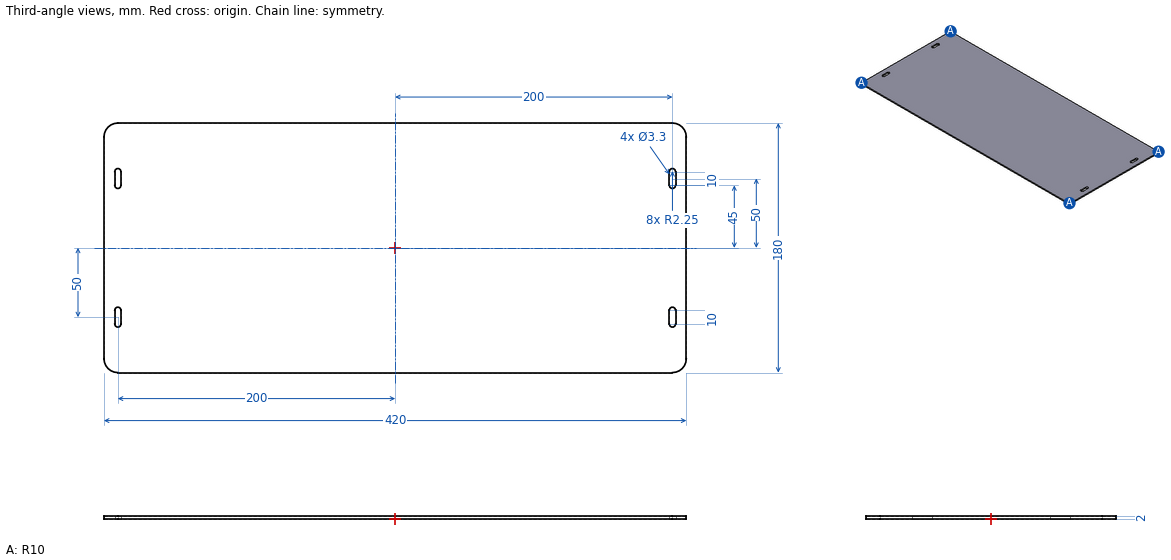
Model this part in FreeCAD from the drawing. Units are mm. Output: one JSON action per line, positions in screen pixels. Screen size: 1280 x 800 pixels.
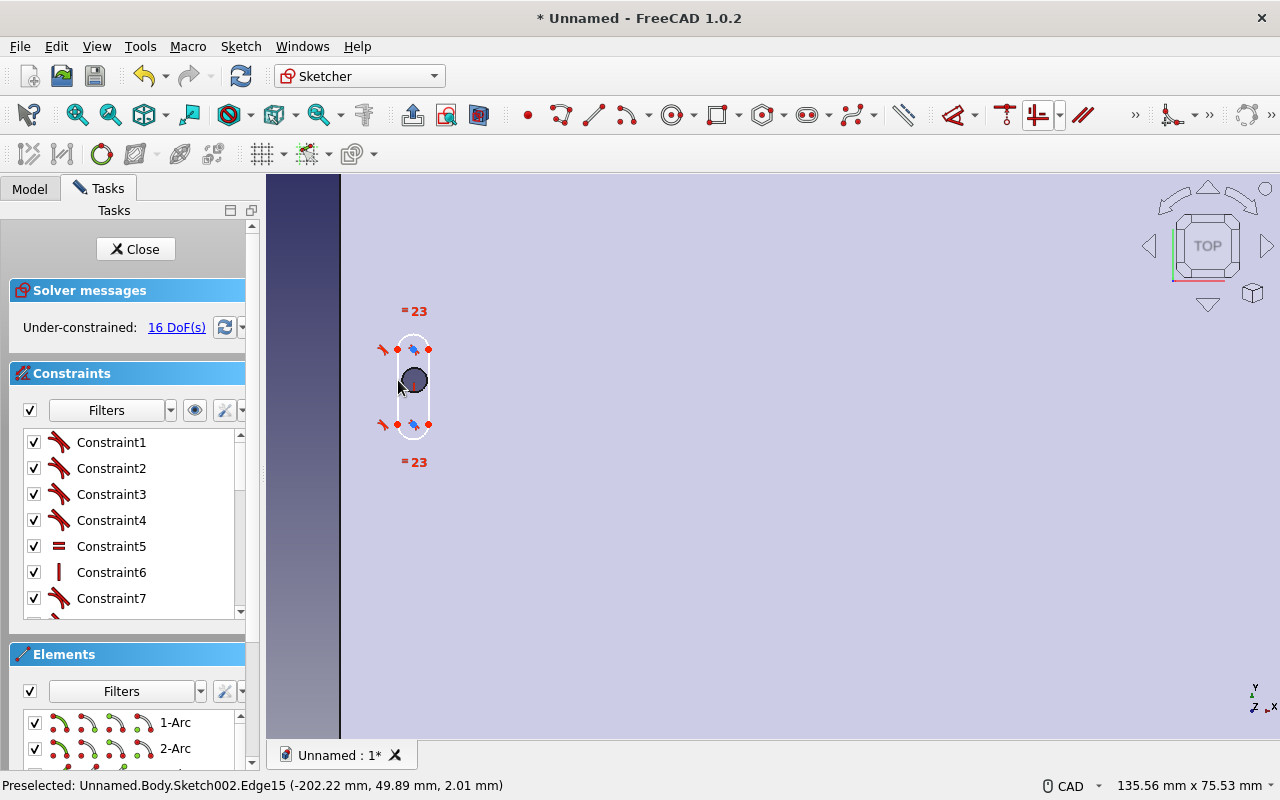
{"action": "scroll", "coordinate": [399, 381], "scroll_direction": "down", "scroll_amount": 8}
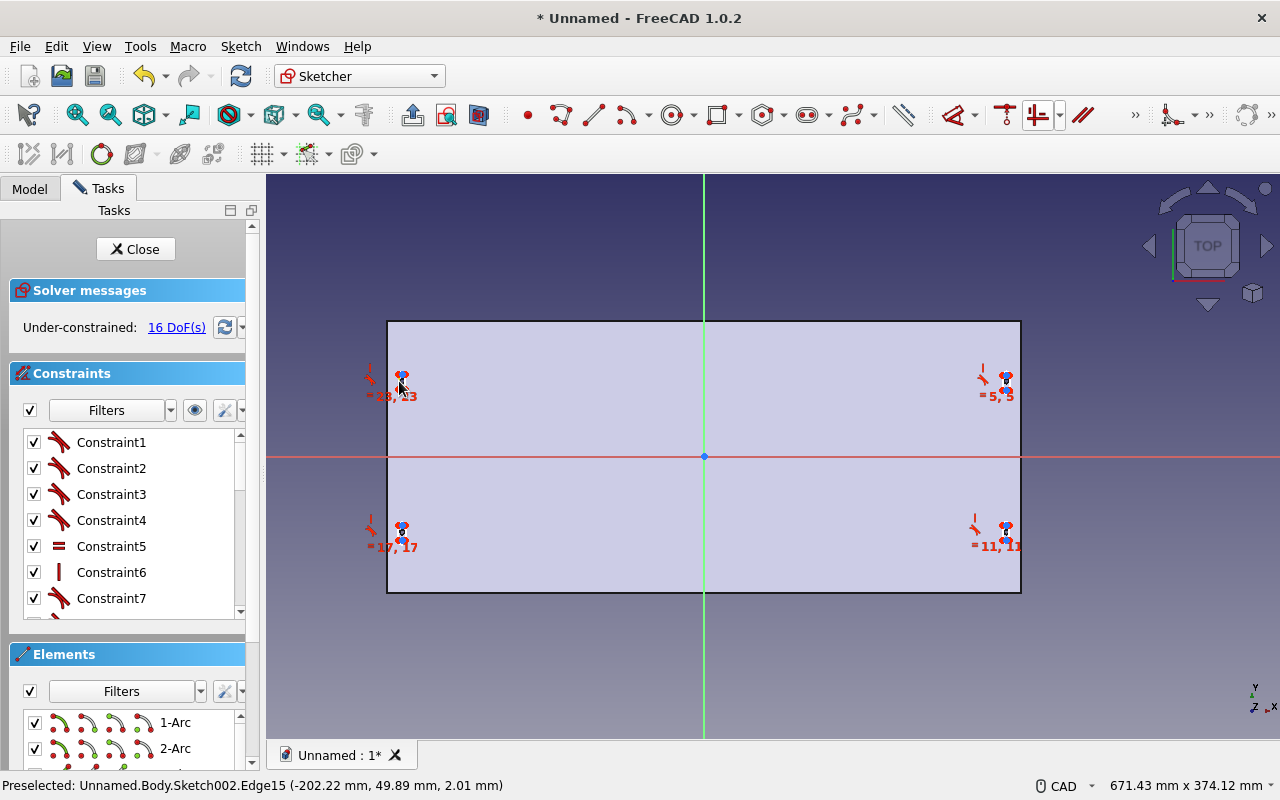
{"action": "scroll", "coordinate": [1004, 393], "scroll_direction": "up", "scroll_amount": 8}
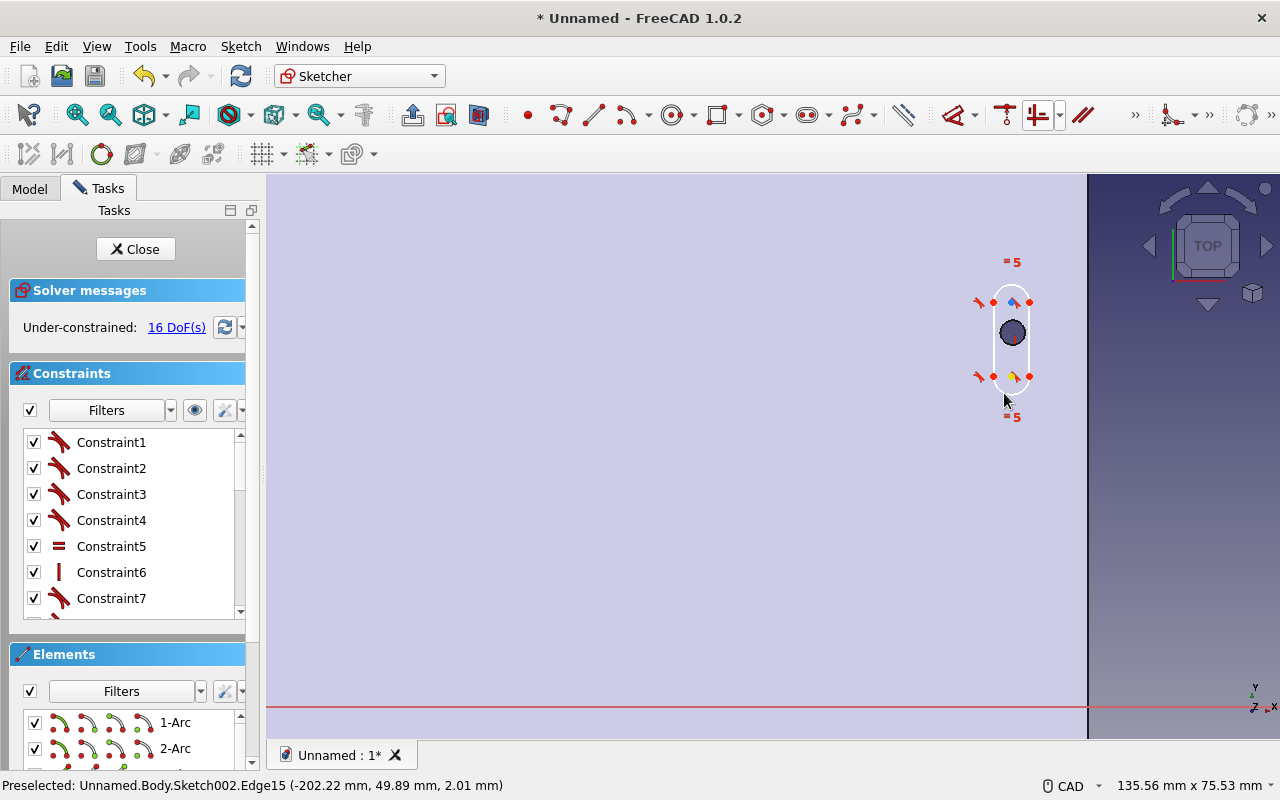
{"action": "left_click", "coordinate": [1001, 391]}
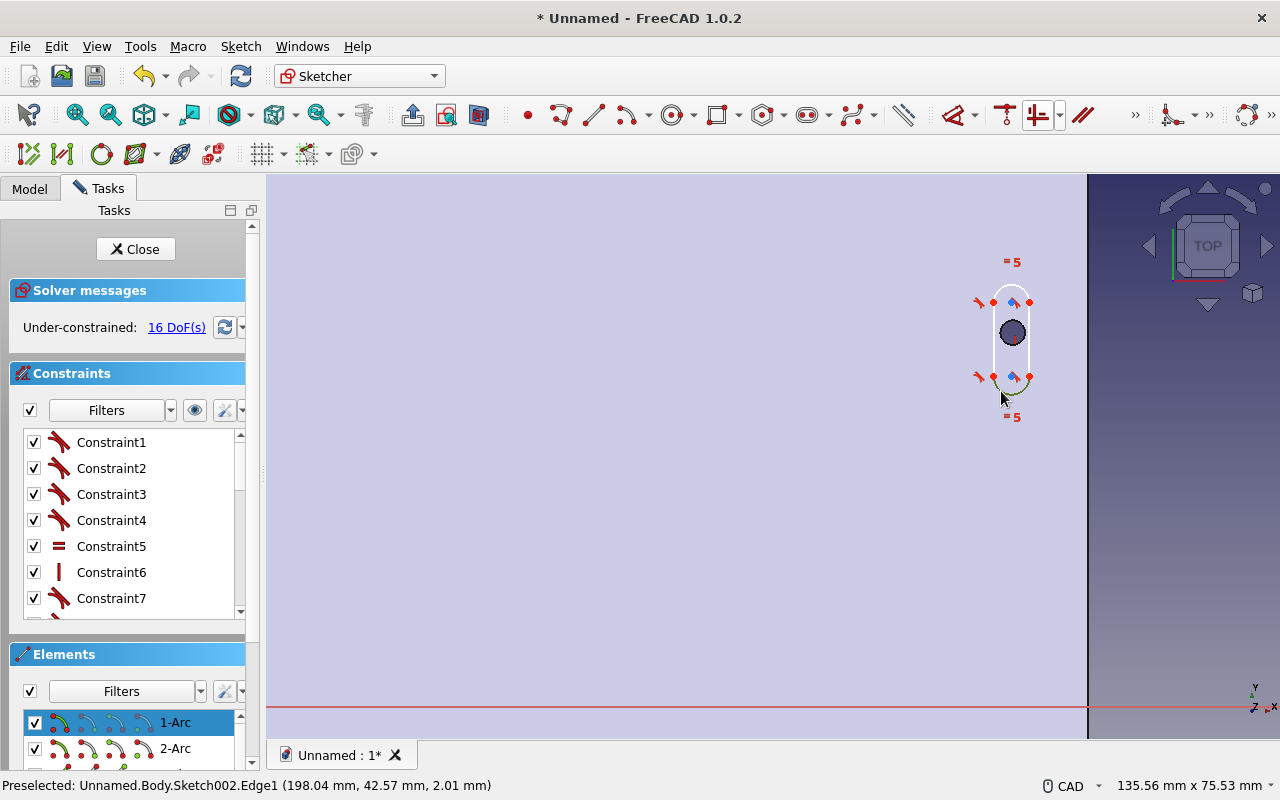
{"action": "scroll", "coordinate": [1005, 393], "scroll_direction": "down", "scroll_amount": 8}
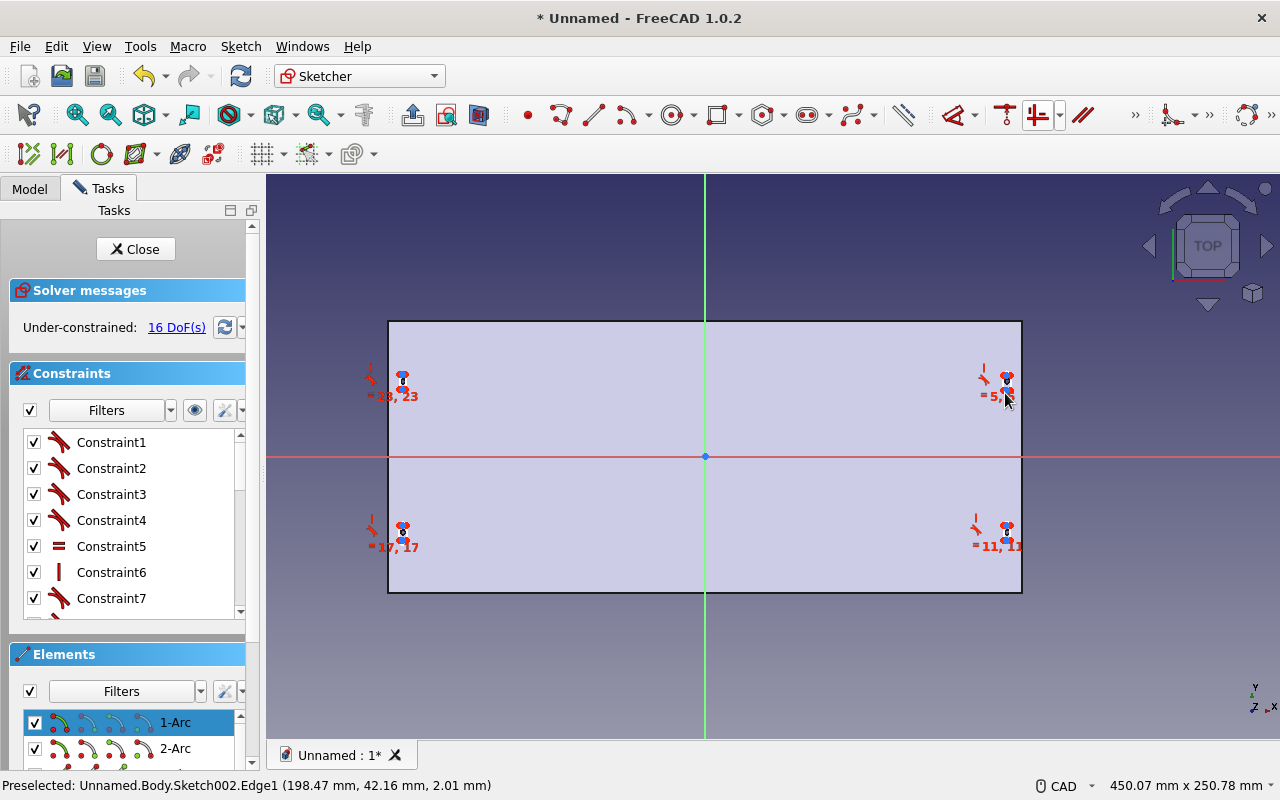
{"action": "scroll", "coordinate": [1005, 543], "scroll_direction": "up", "scroll_amount": 8}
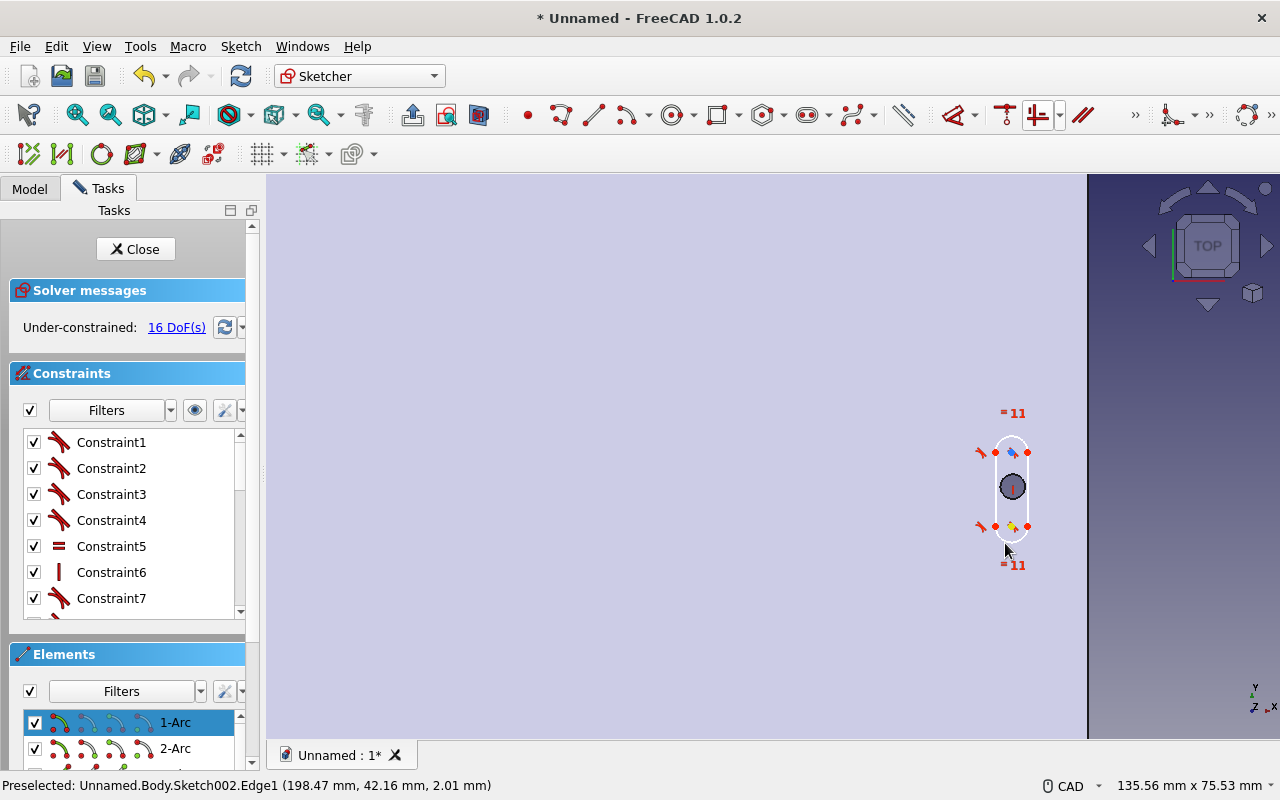
{"action": "left_click", "coordinate": [1002, 539]}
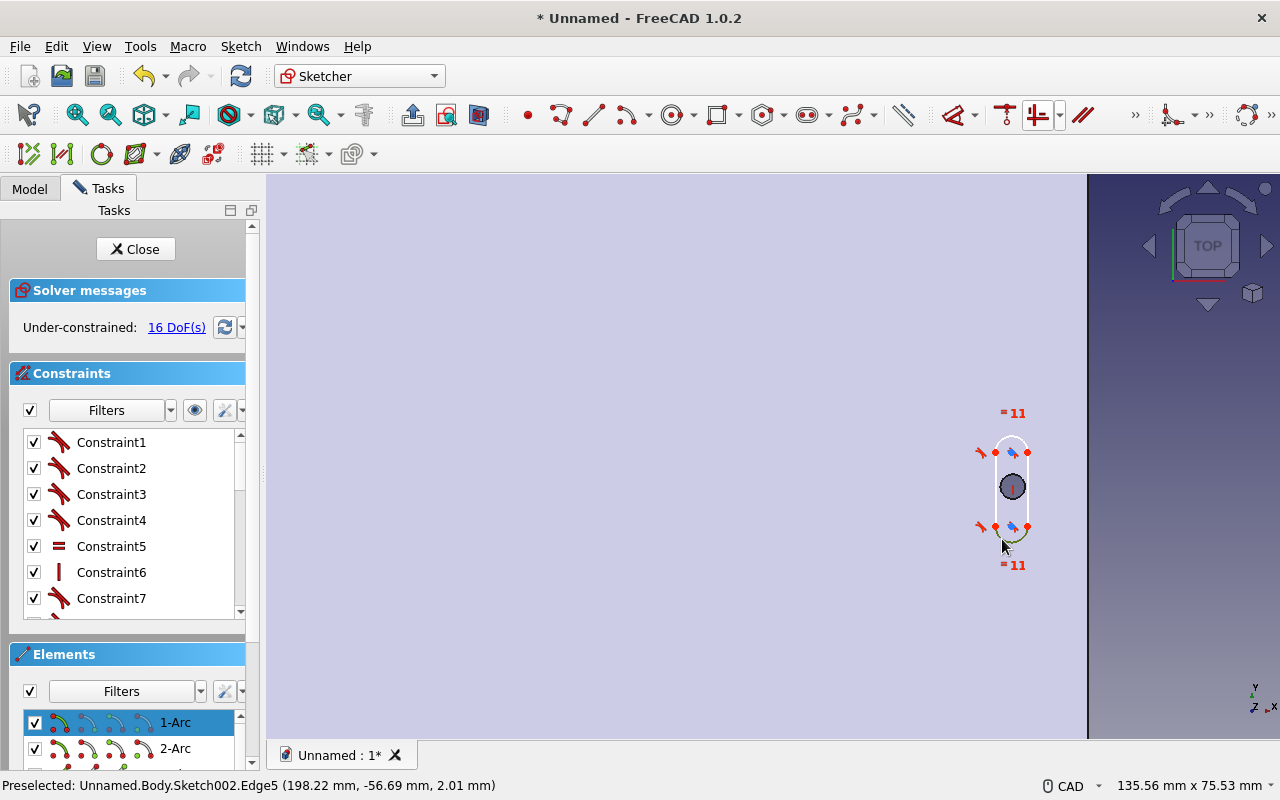
{"action": "scroll", "coordinate": [1005, 543], "scroll_direction": "down", "scroll_amount": 8}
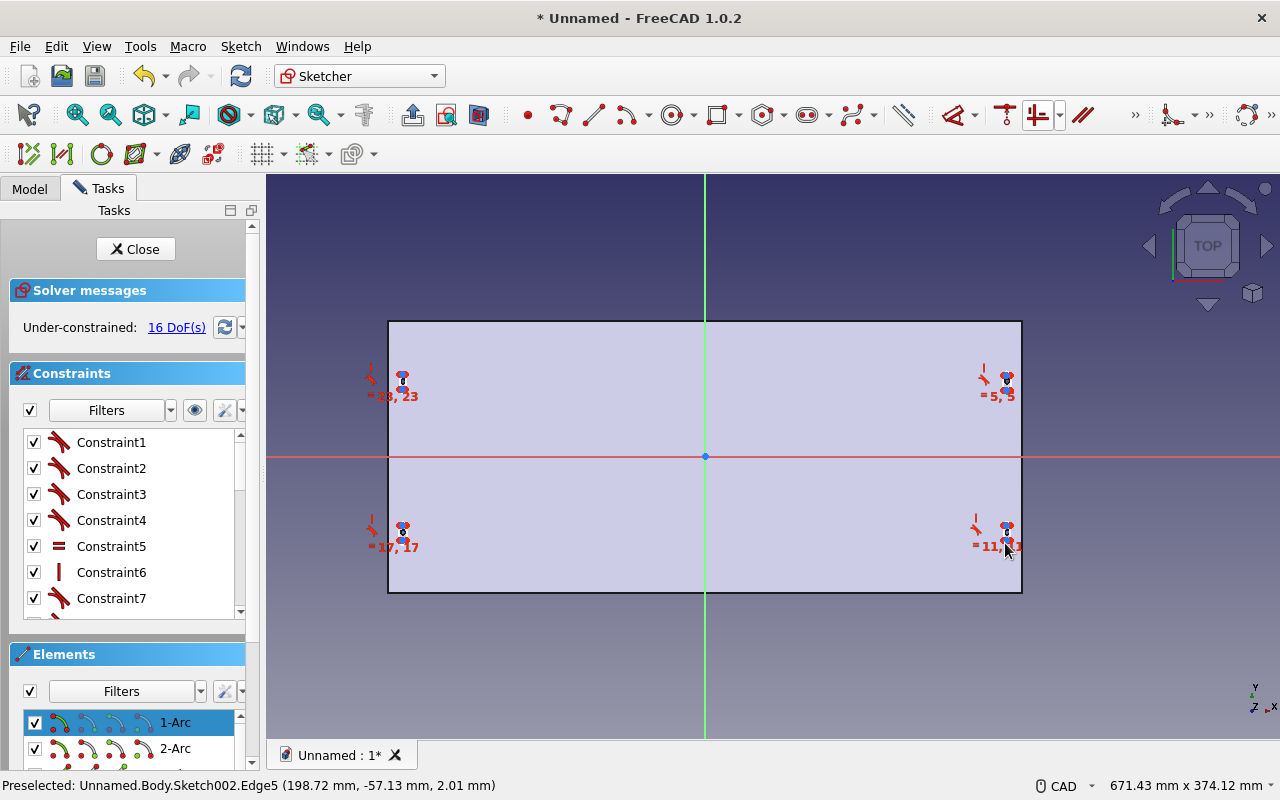
{"action": "scroll", "coordinate": [401, 544], "scroll_direction": "up", "scroll_amount": 8}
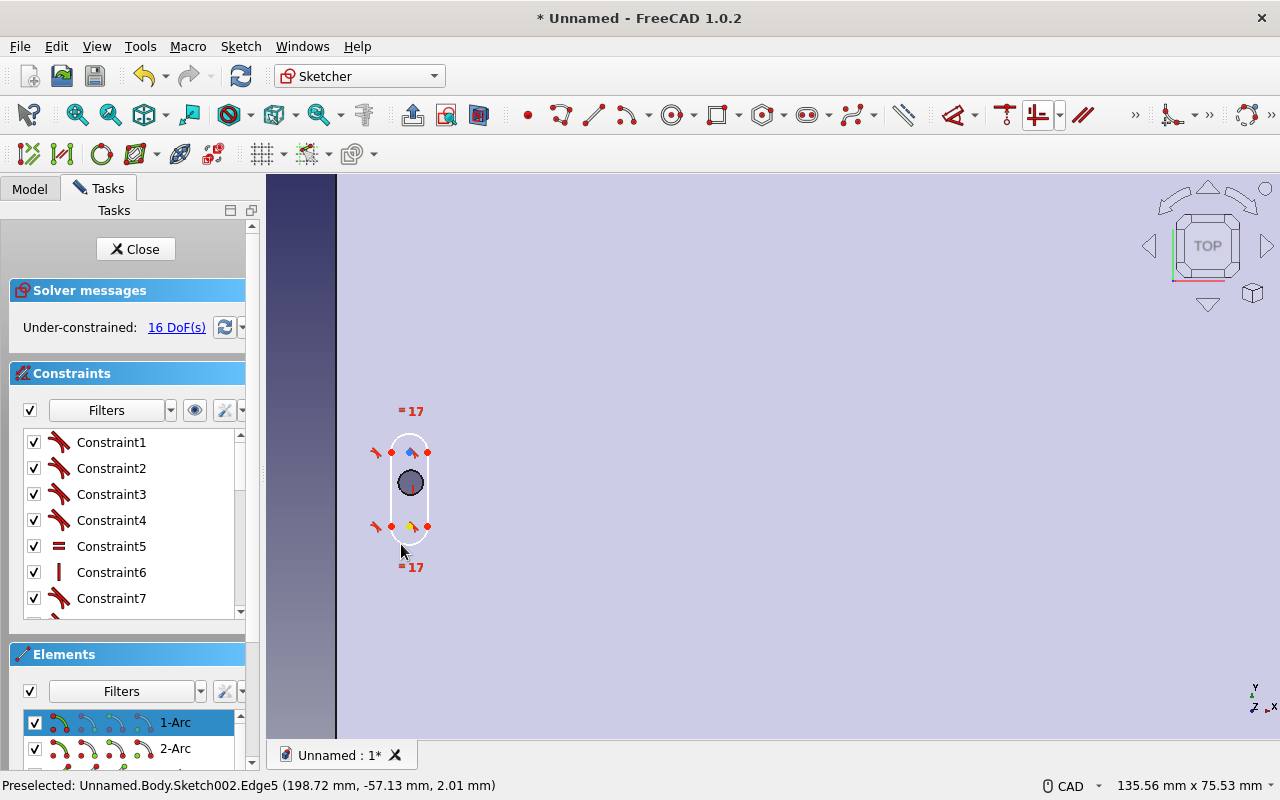
{"action": "left_click", "coordinate": [399, 541]}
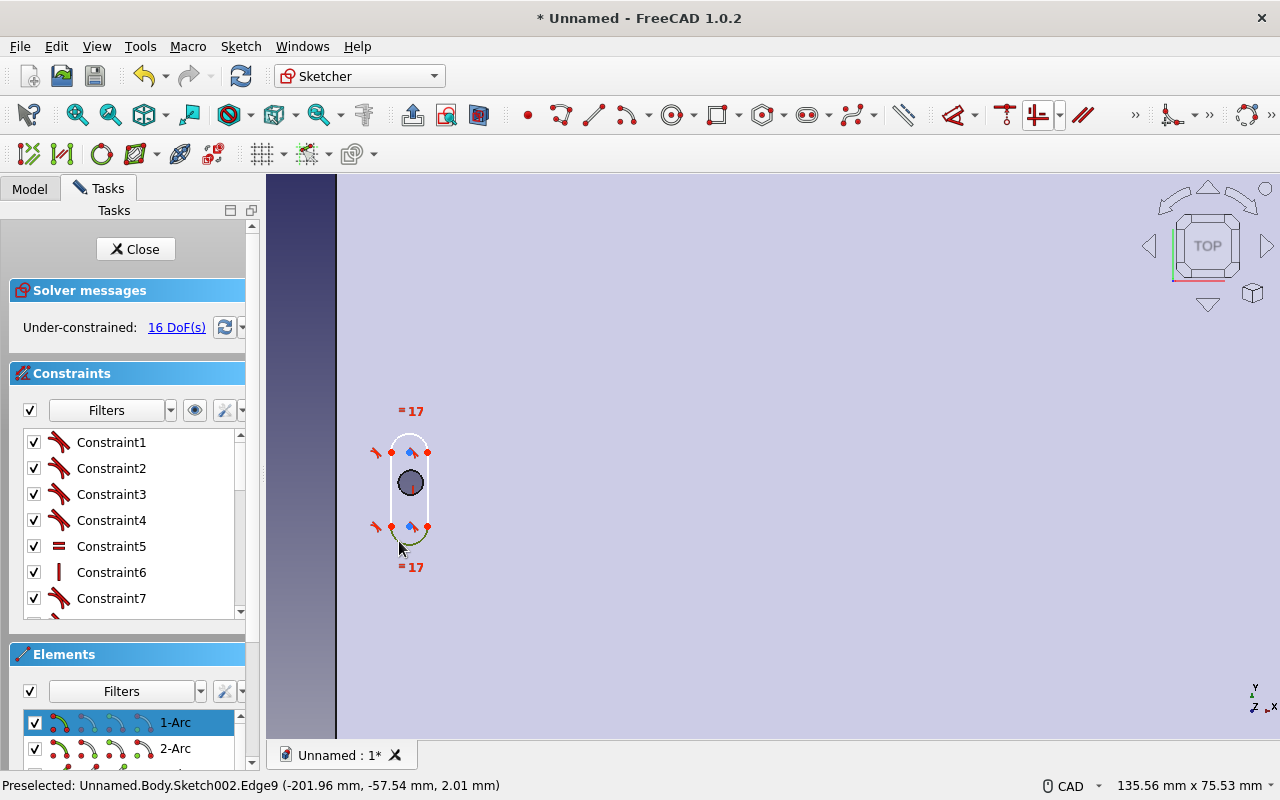
{"action": "scroll", "coordinate": [400, 544], "scroll_direction": "down", "scroll_amount": 8}